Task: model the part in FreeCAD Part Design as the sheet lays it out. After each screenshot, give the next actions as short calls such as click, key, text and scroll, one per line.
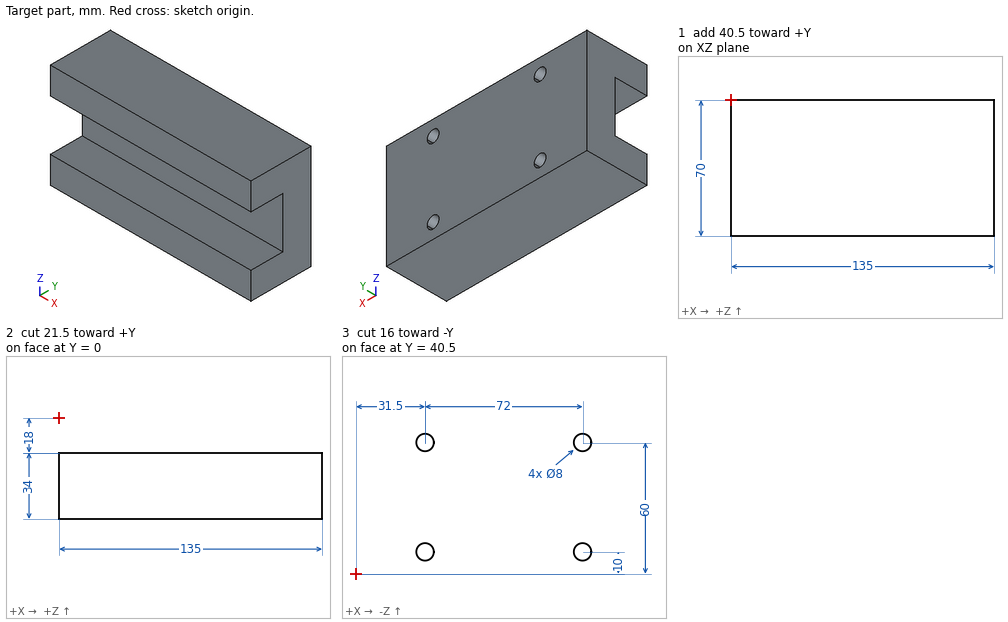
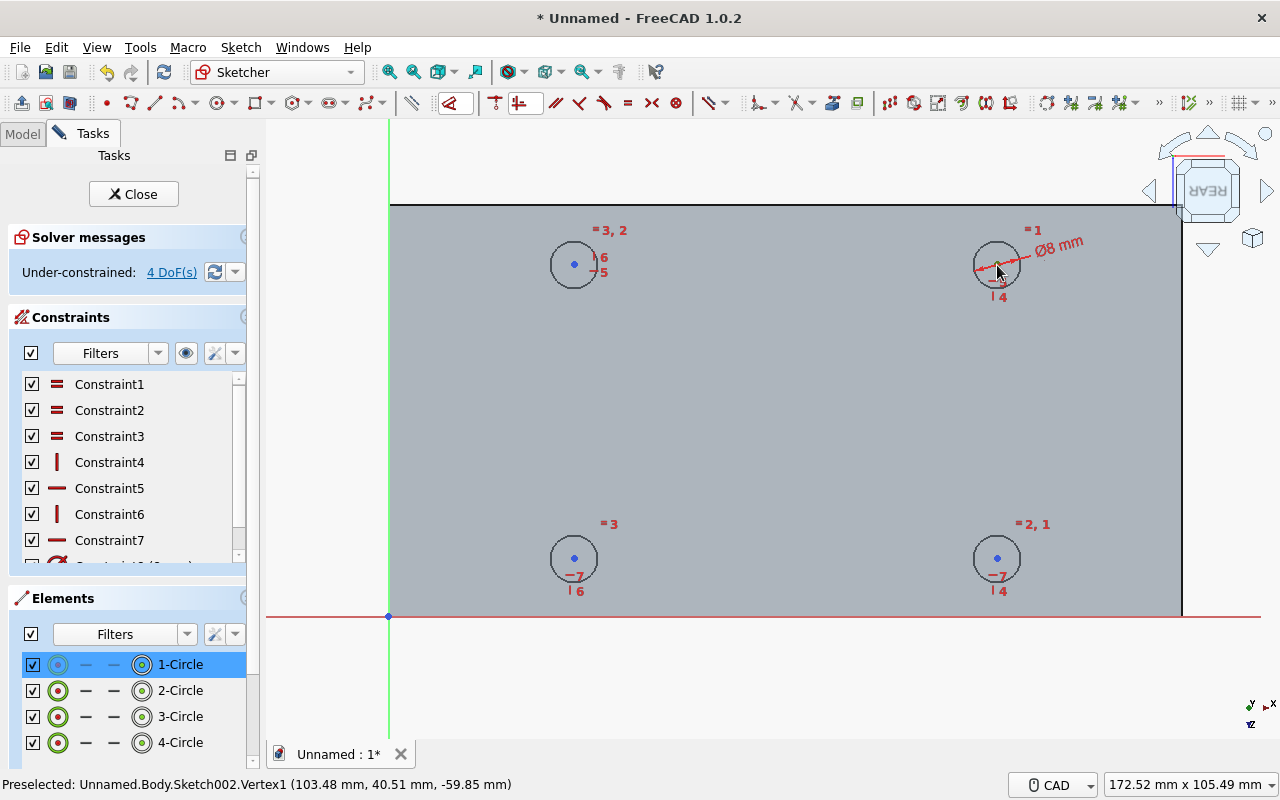
click(468, 104)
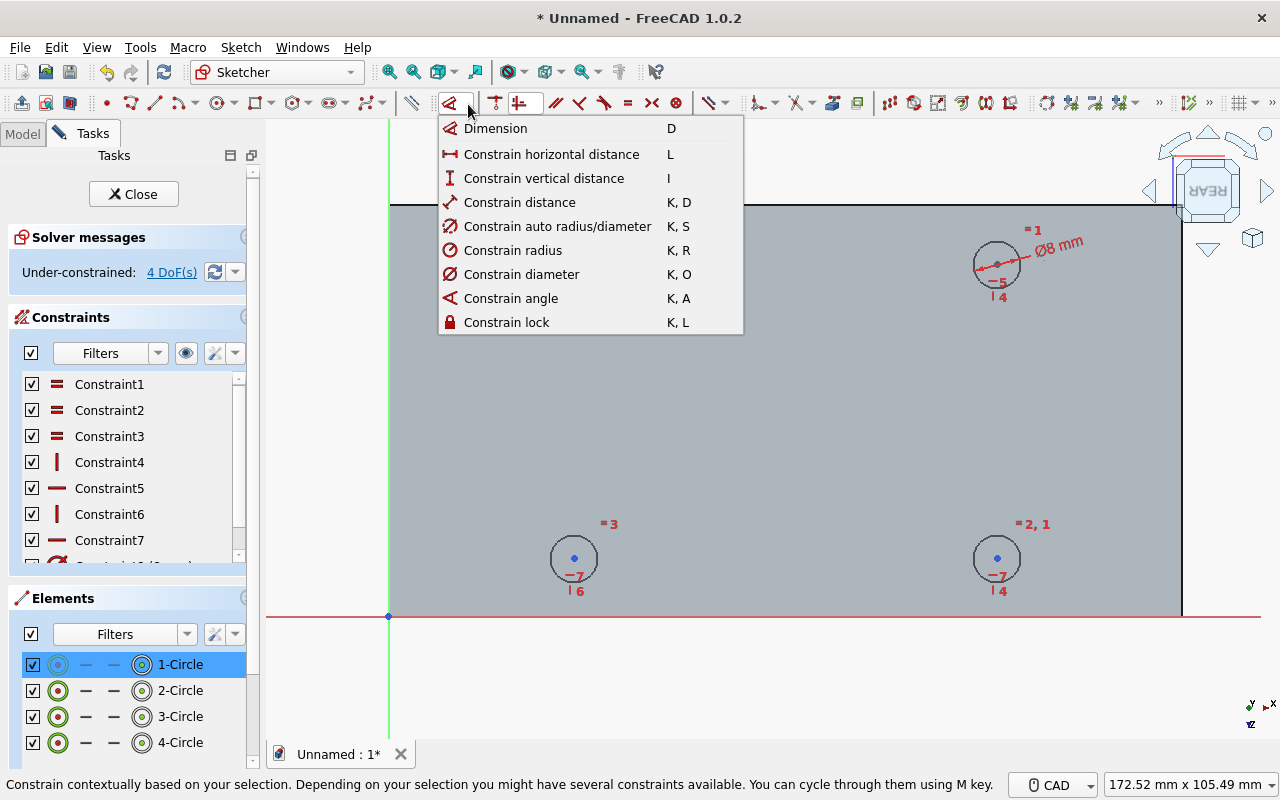
click(591, 178)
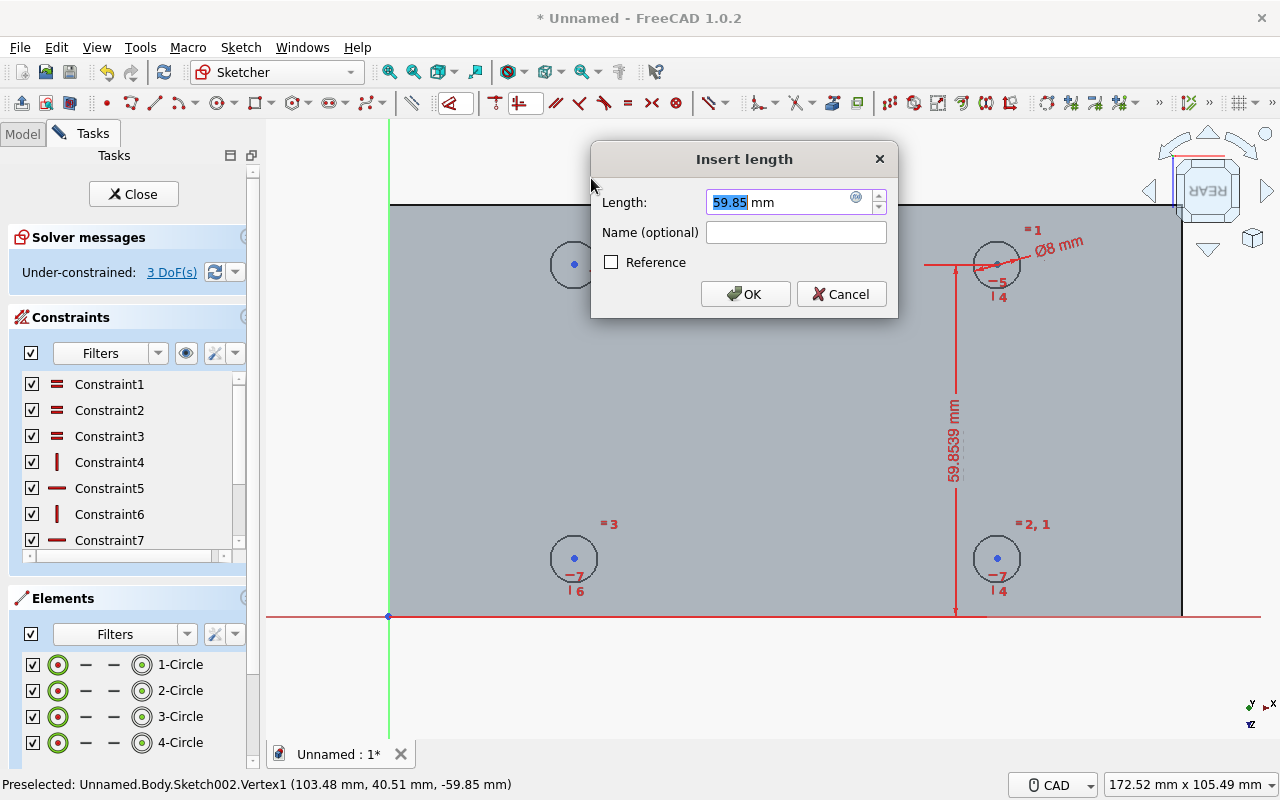
text(60)
key(Return)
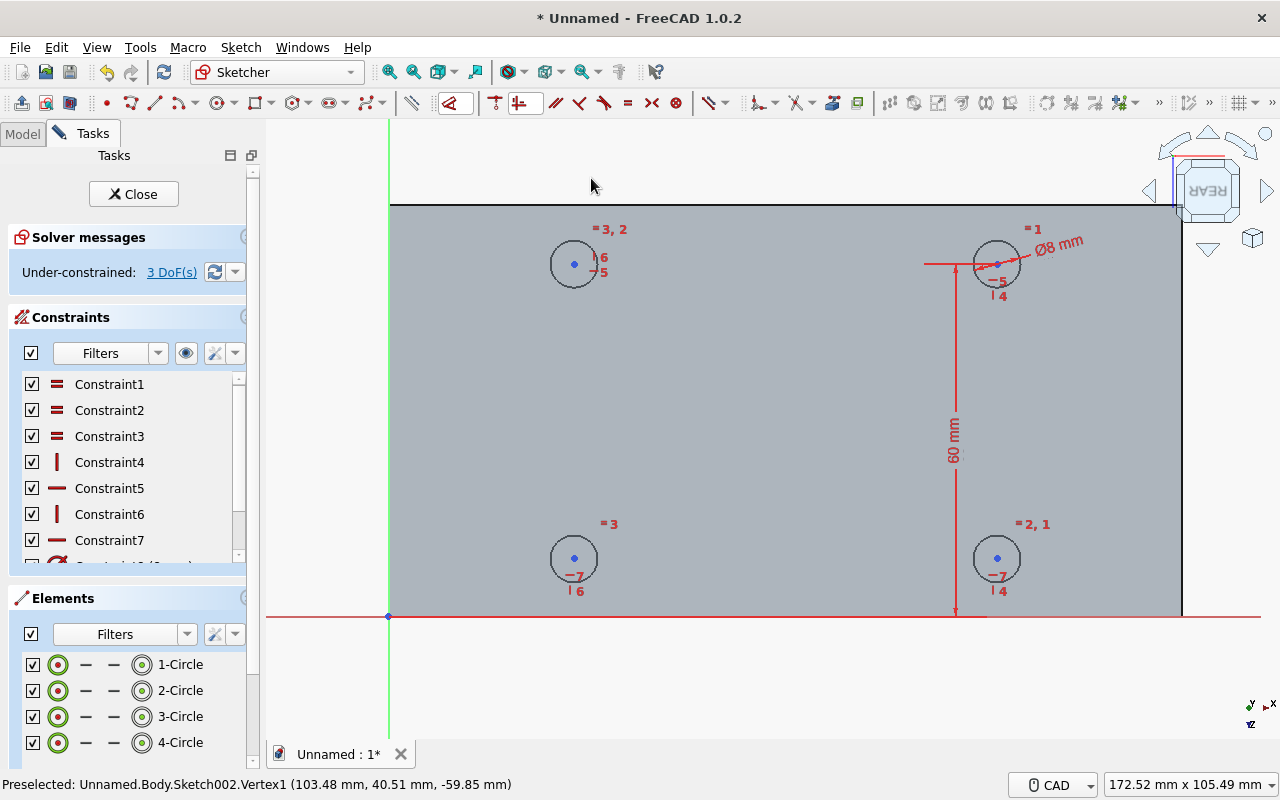
click(997, 559)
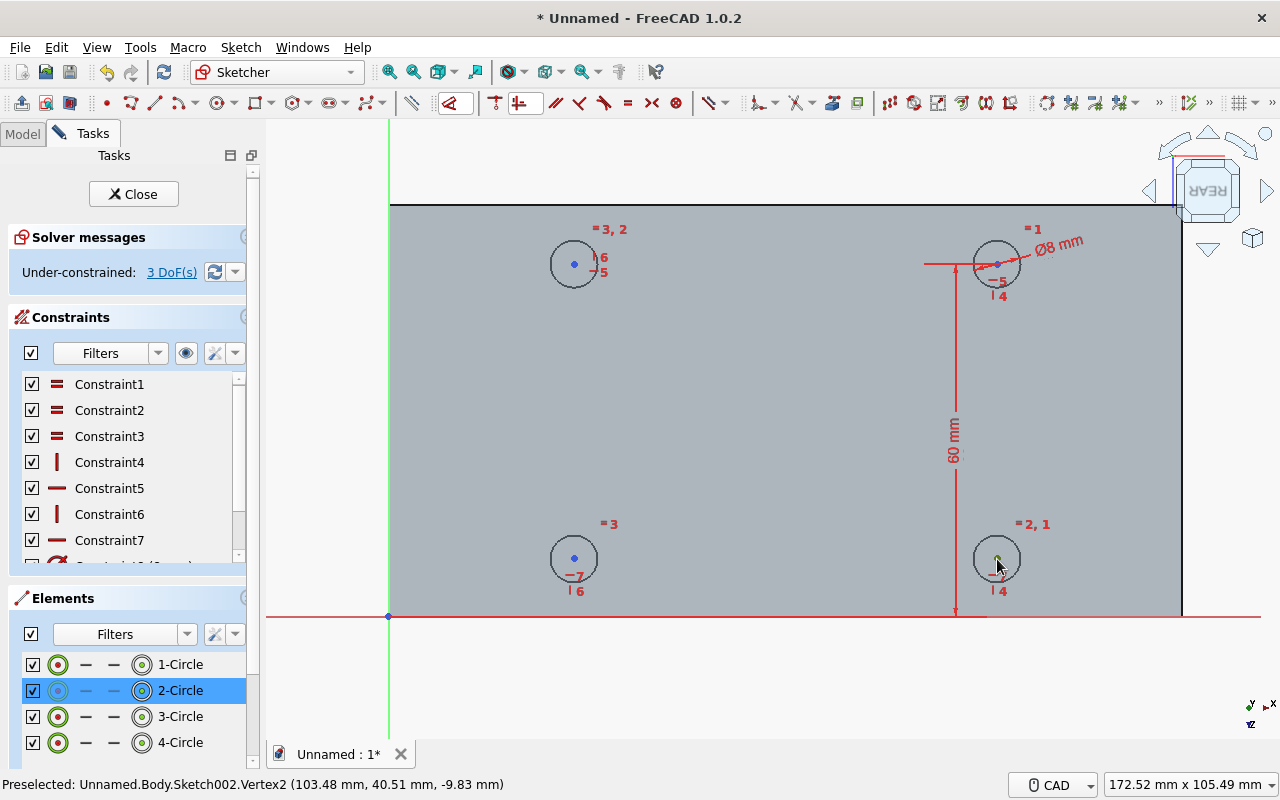
click(468, 104)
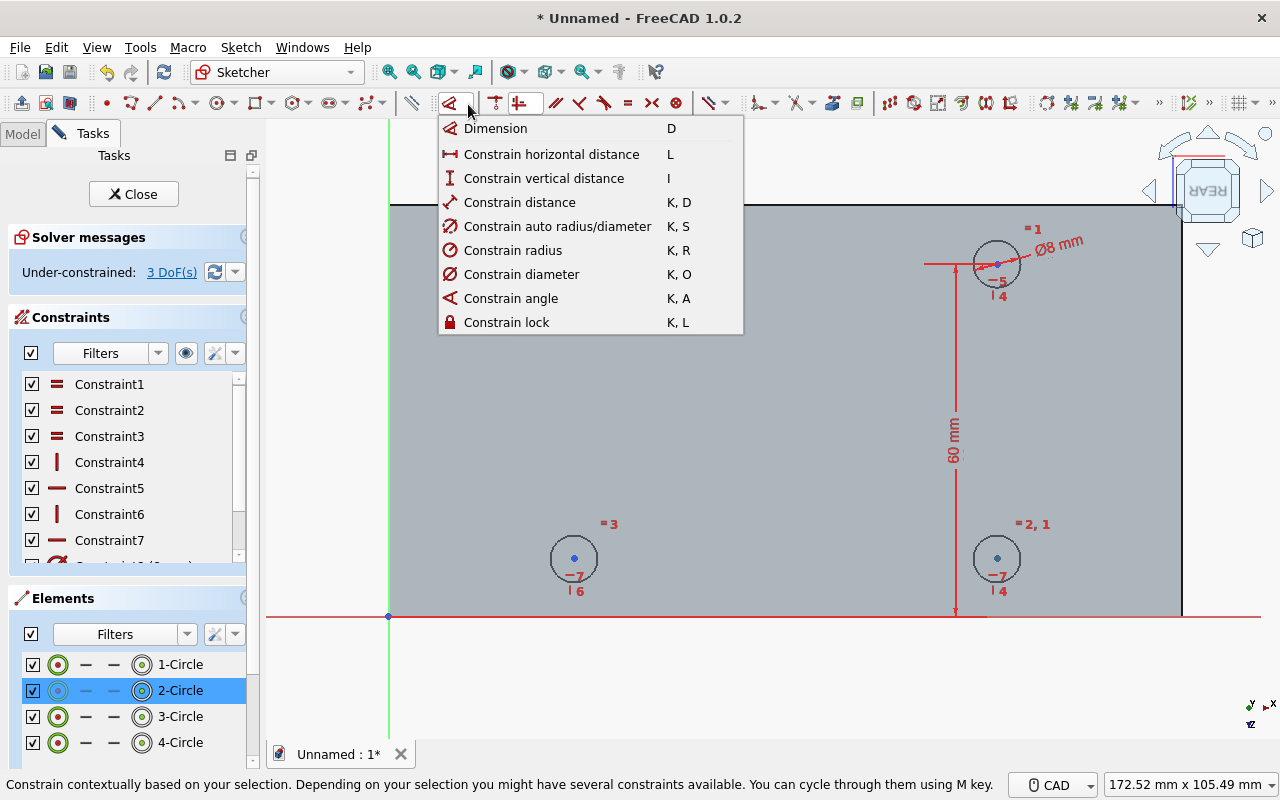
click(591, 178)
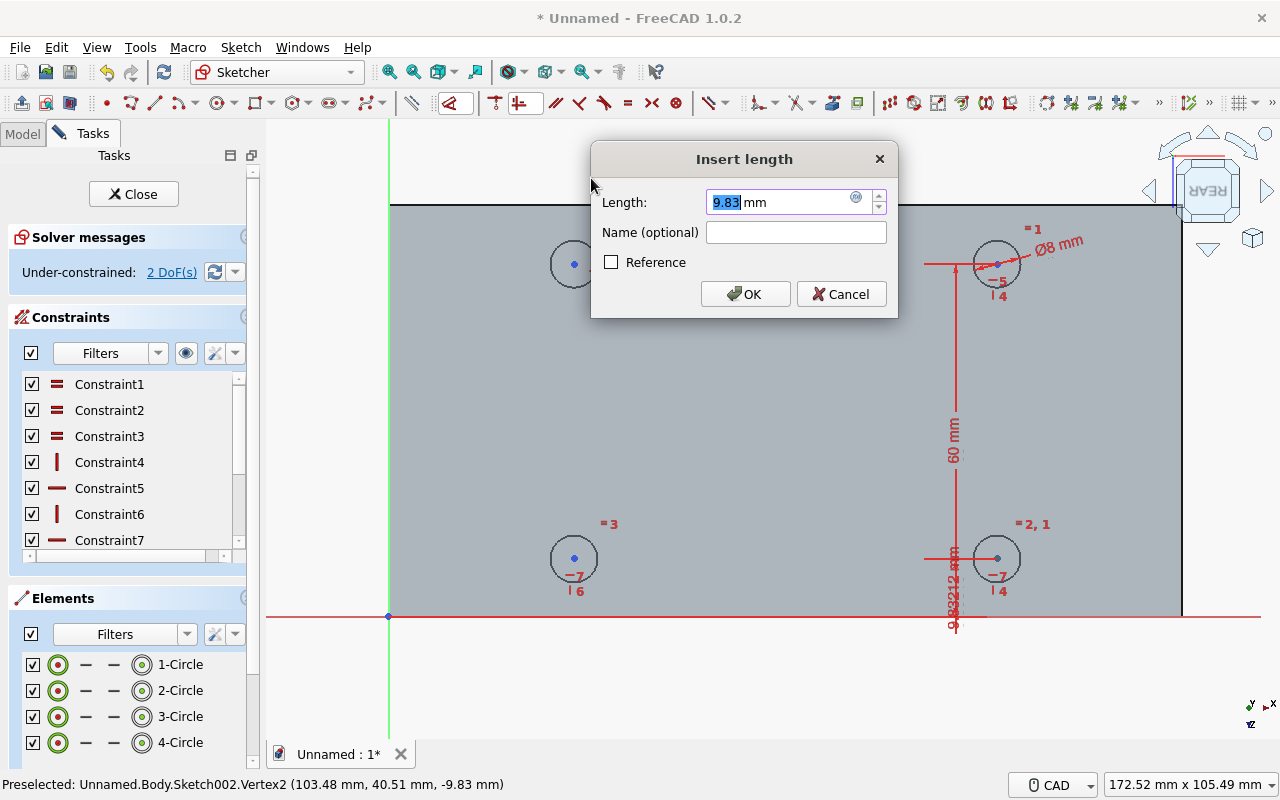
text(10)
key(Return)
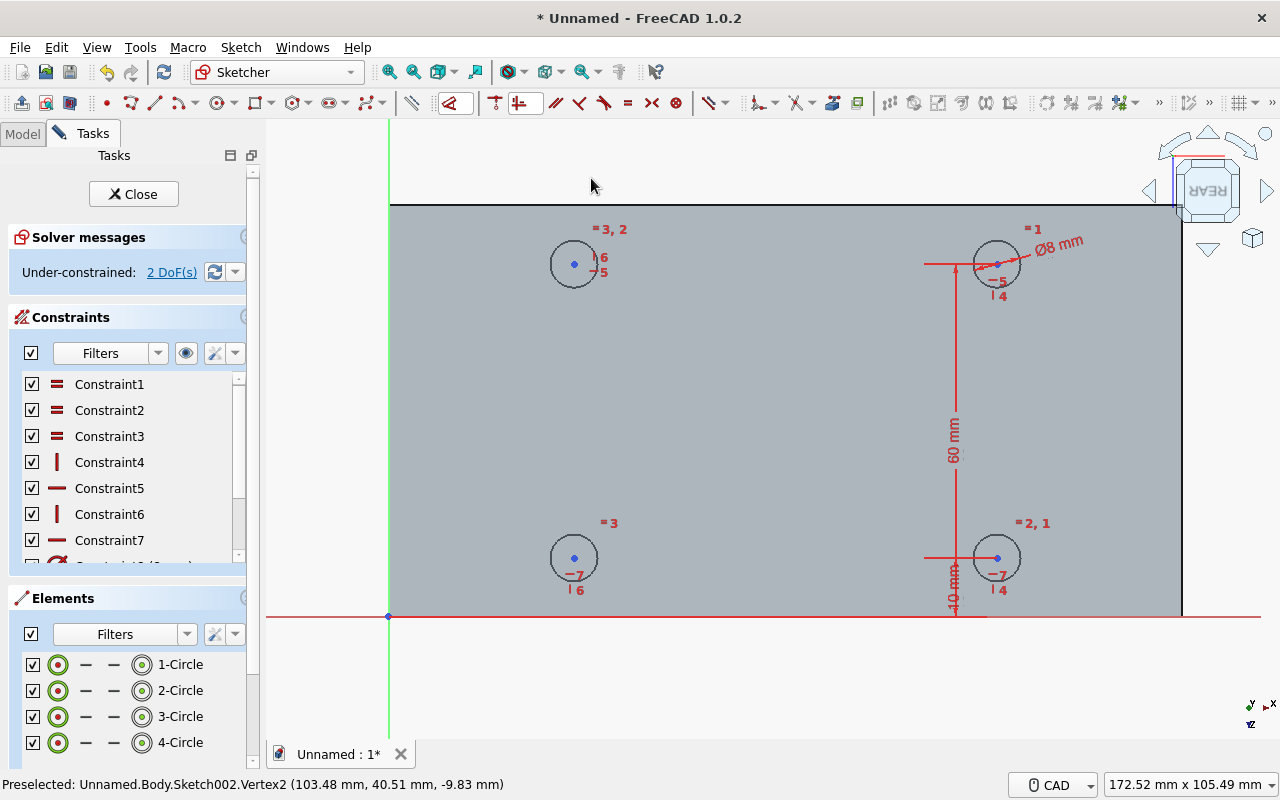
click(997, 264)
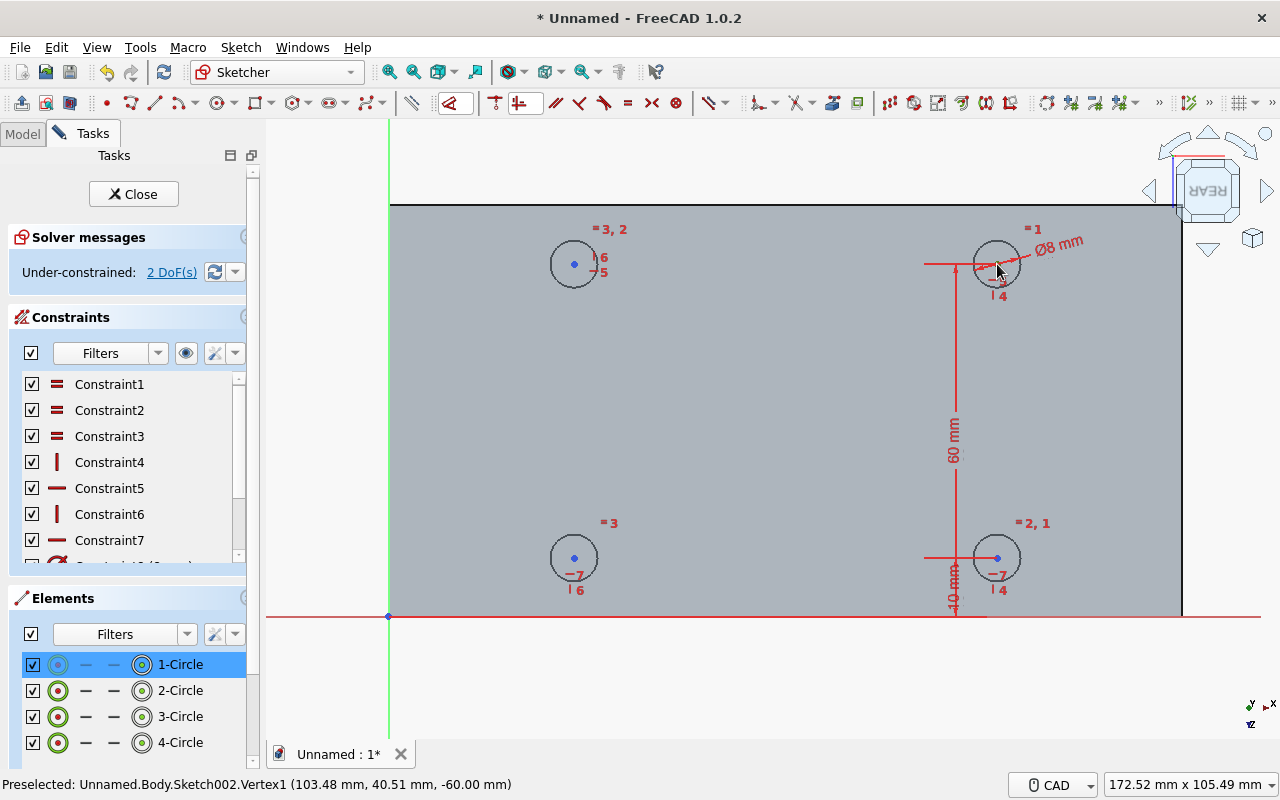
click(574, 264)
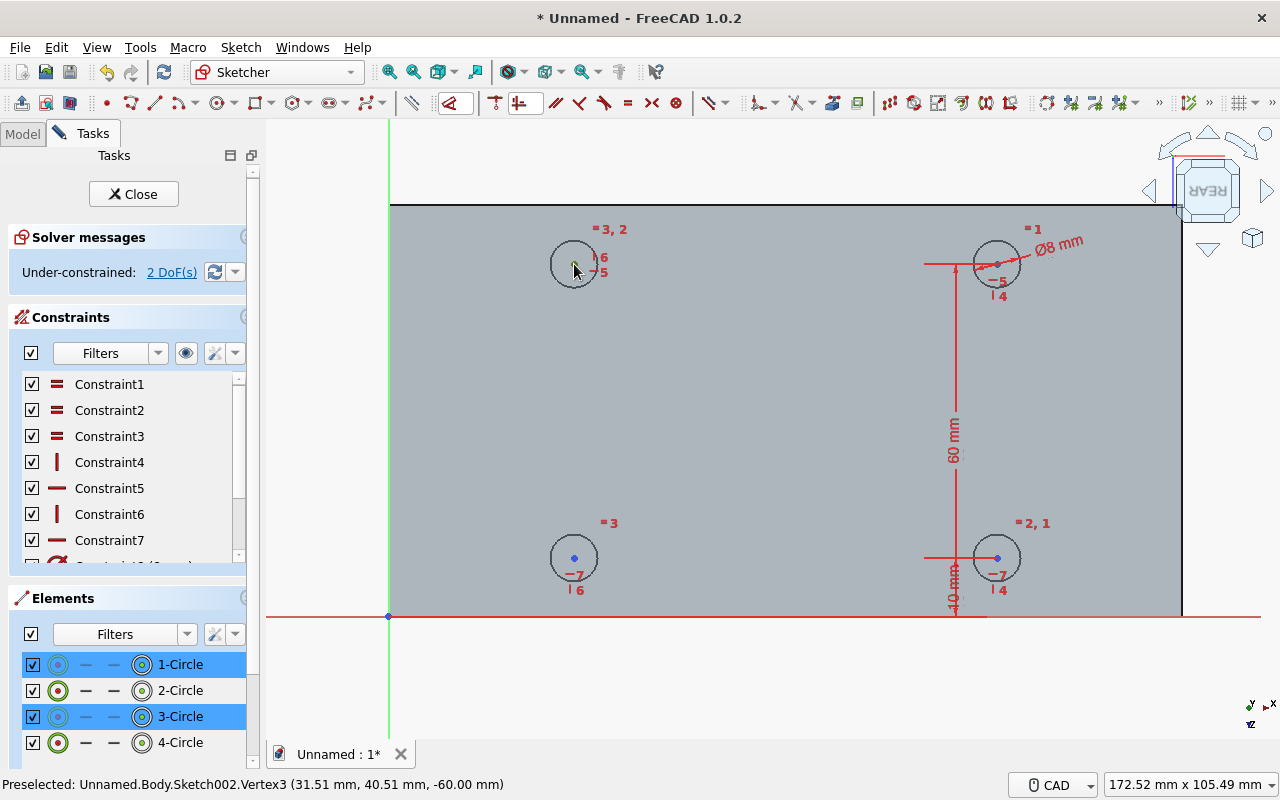
click(468, 104)